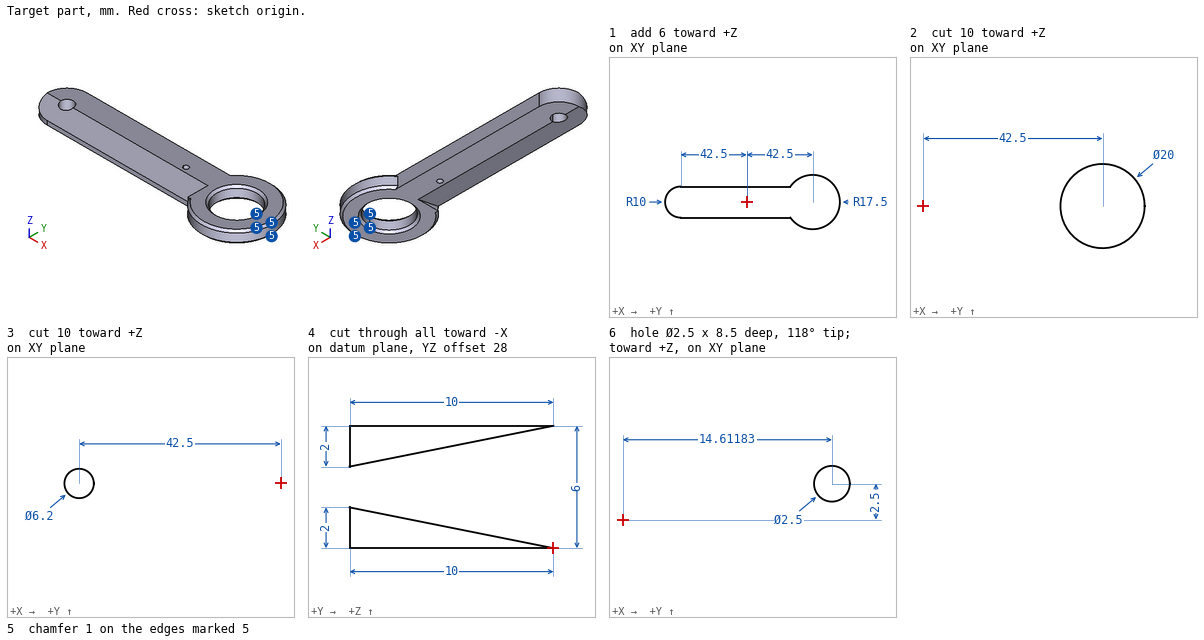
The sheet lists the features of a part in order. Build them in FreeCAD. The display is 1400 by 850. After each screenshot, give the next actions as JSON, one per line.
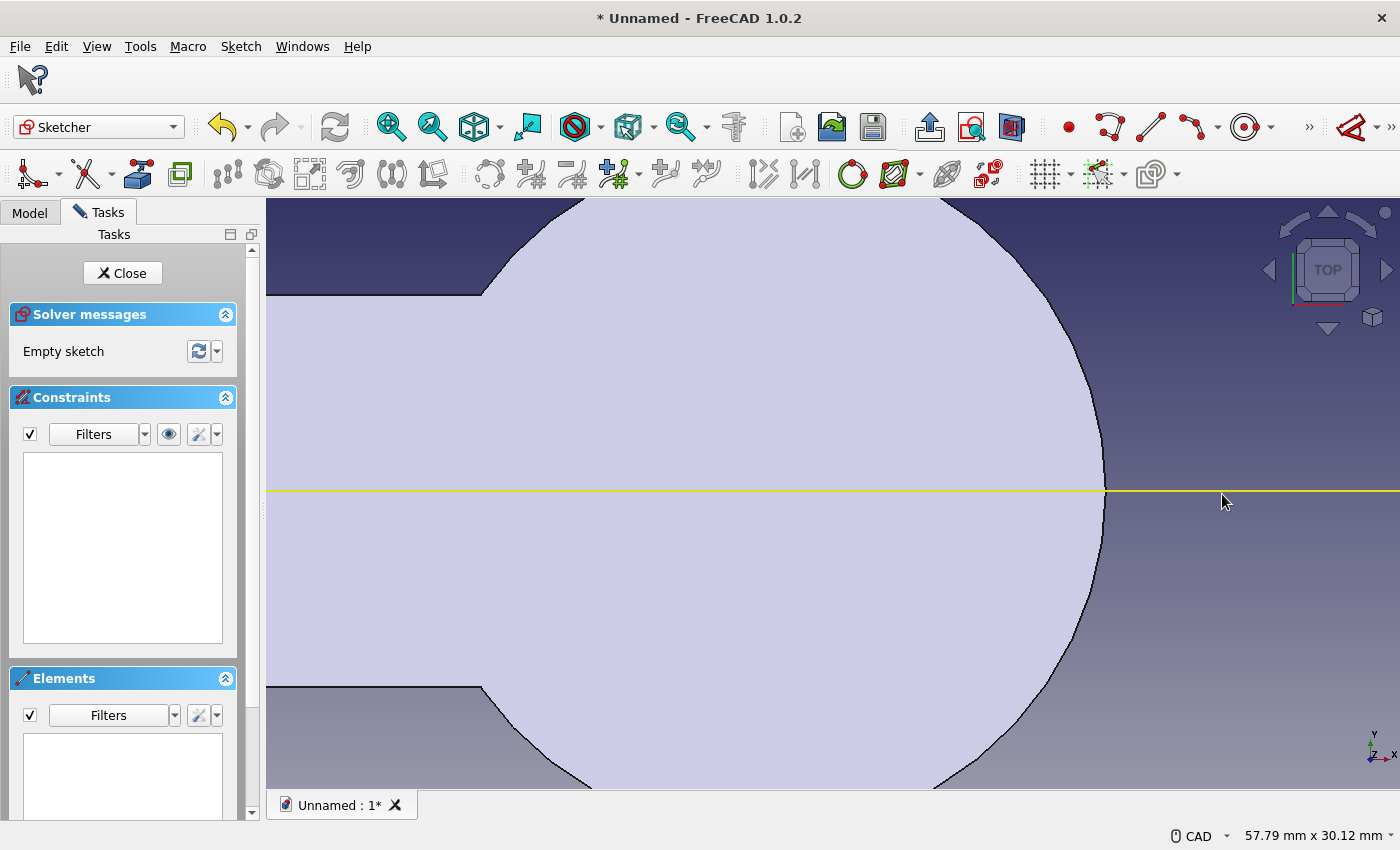
{"action": "key", "text": "g c"}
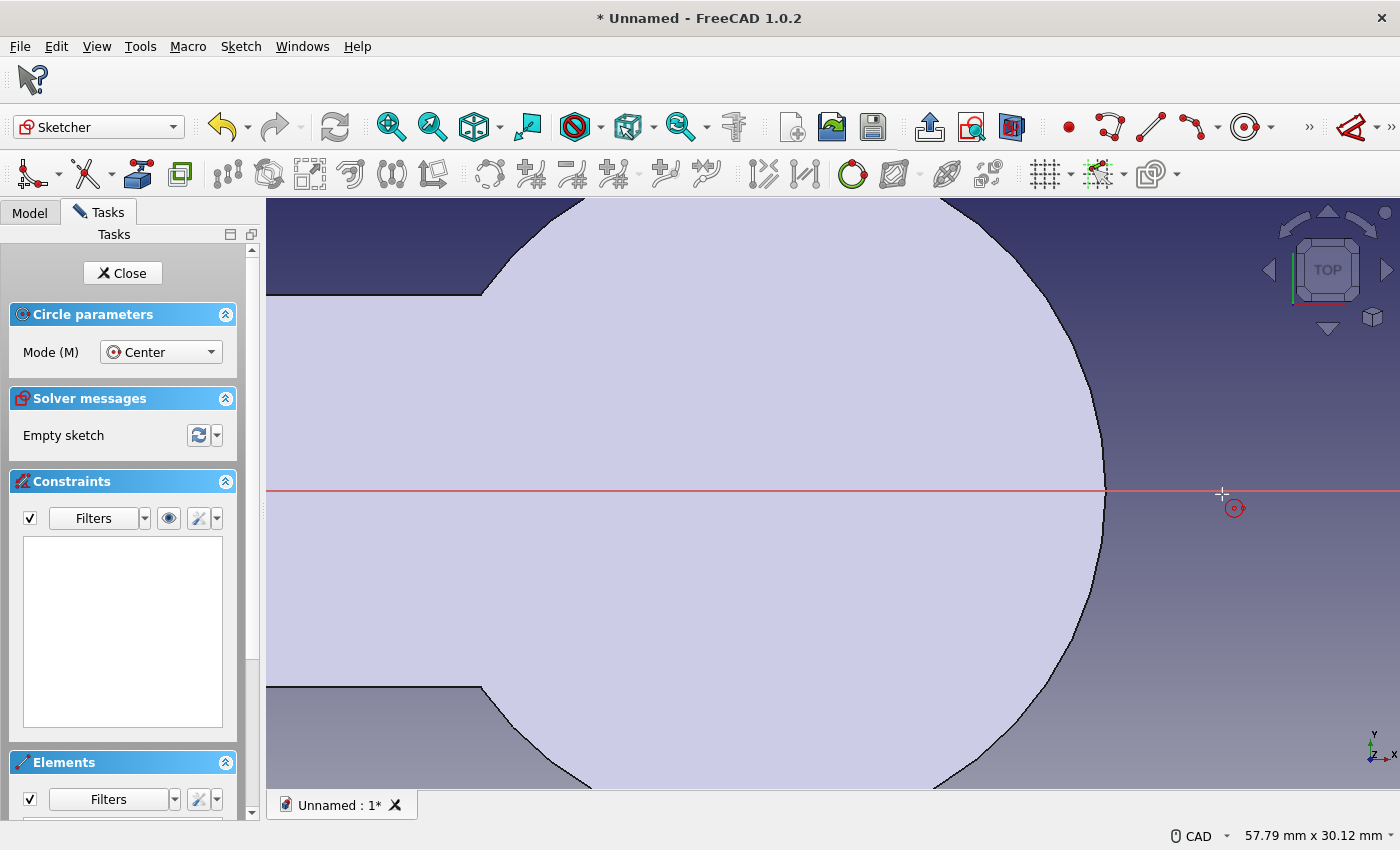
{"action": "left_click", "coordinate": [762, 491]}
{"action": "left_click", "coordinate": [901, 352]}
{"action": "key", "text": "Escape"}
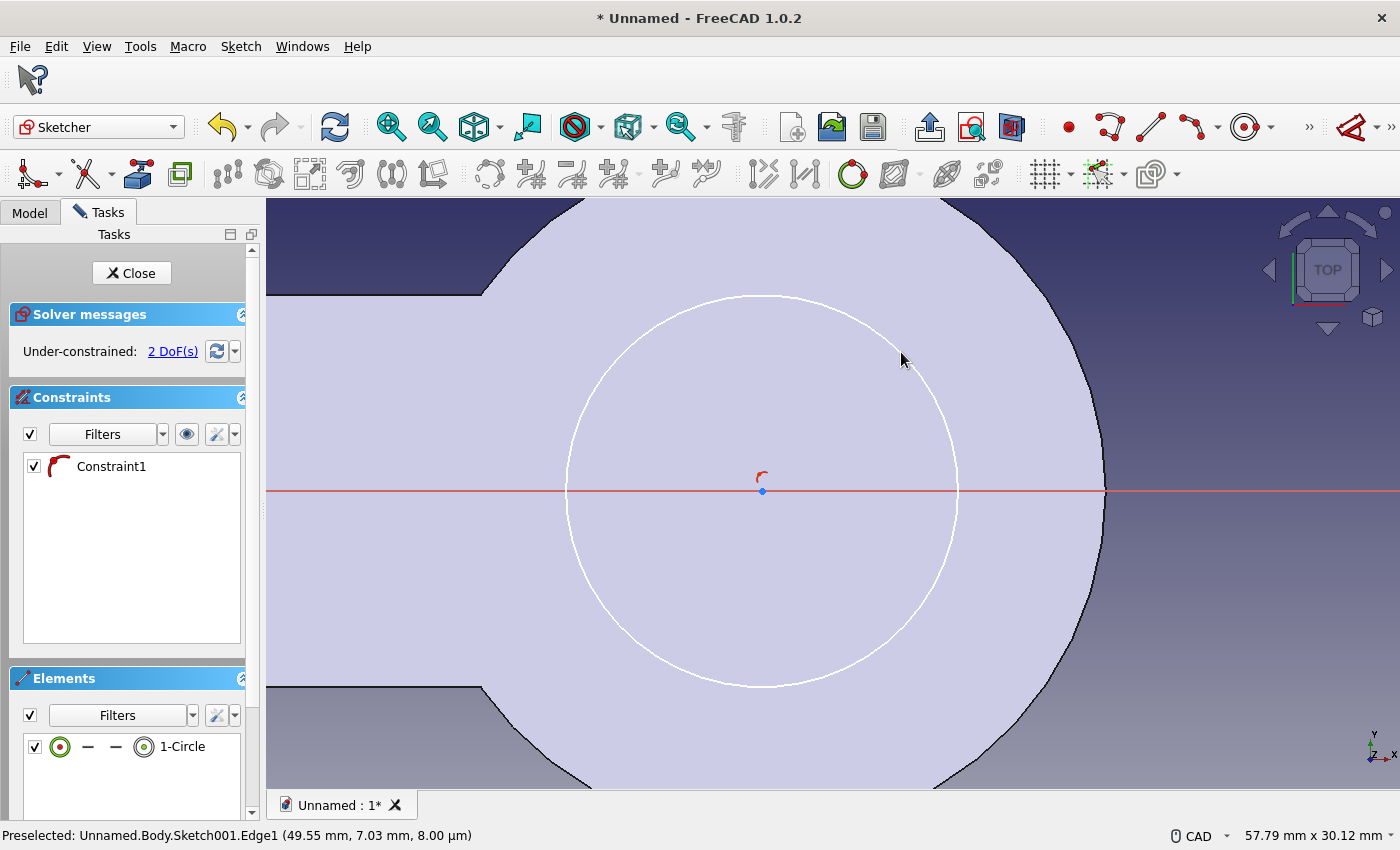
{"action": "left_click", "coordinate": [1350, 128]}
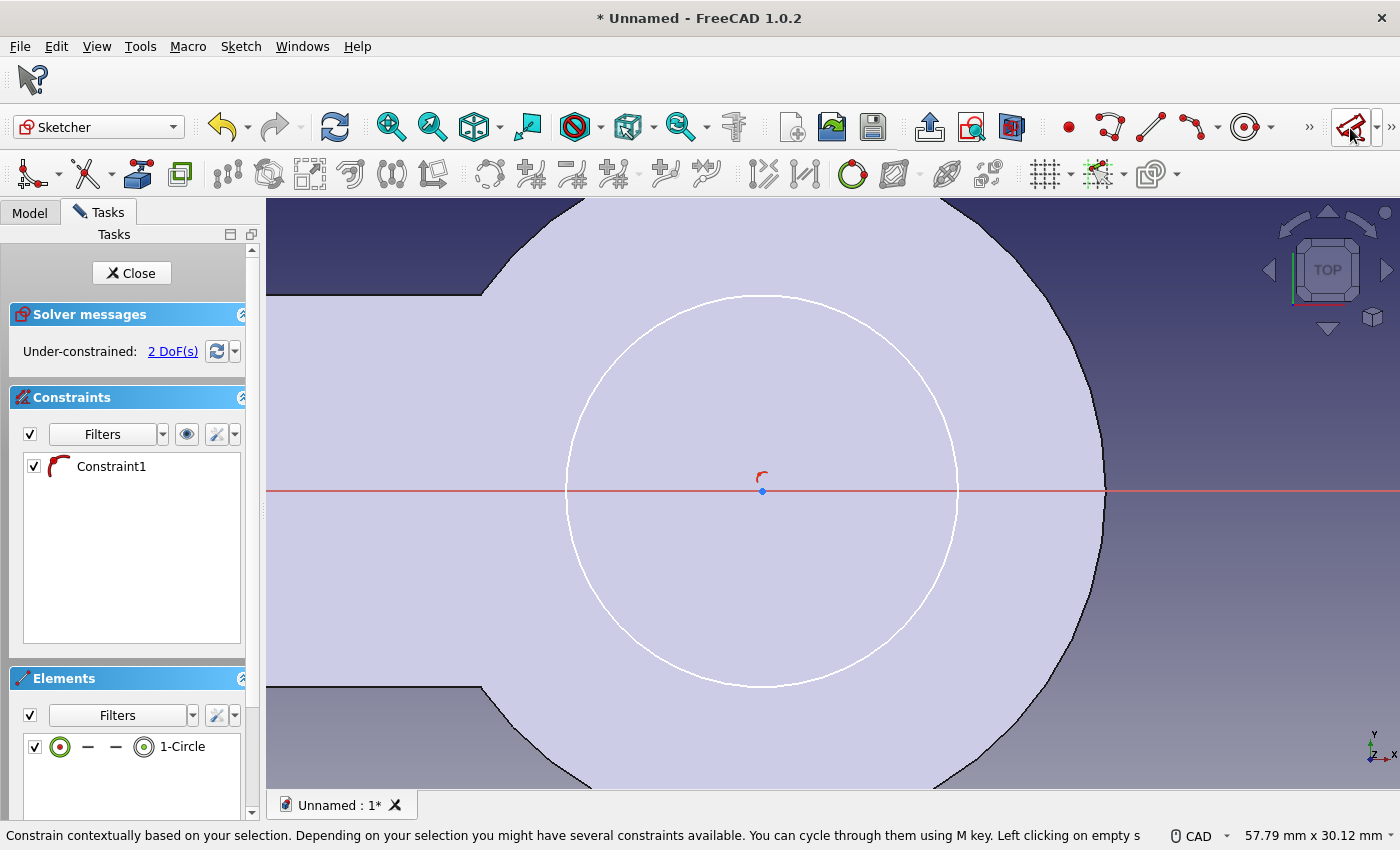
{"action": "left_click", "coordinate": [900, 352]}
{"action": "left_click", "coordinate": [923, 329]}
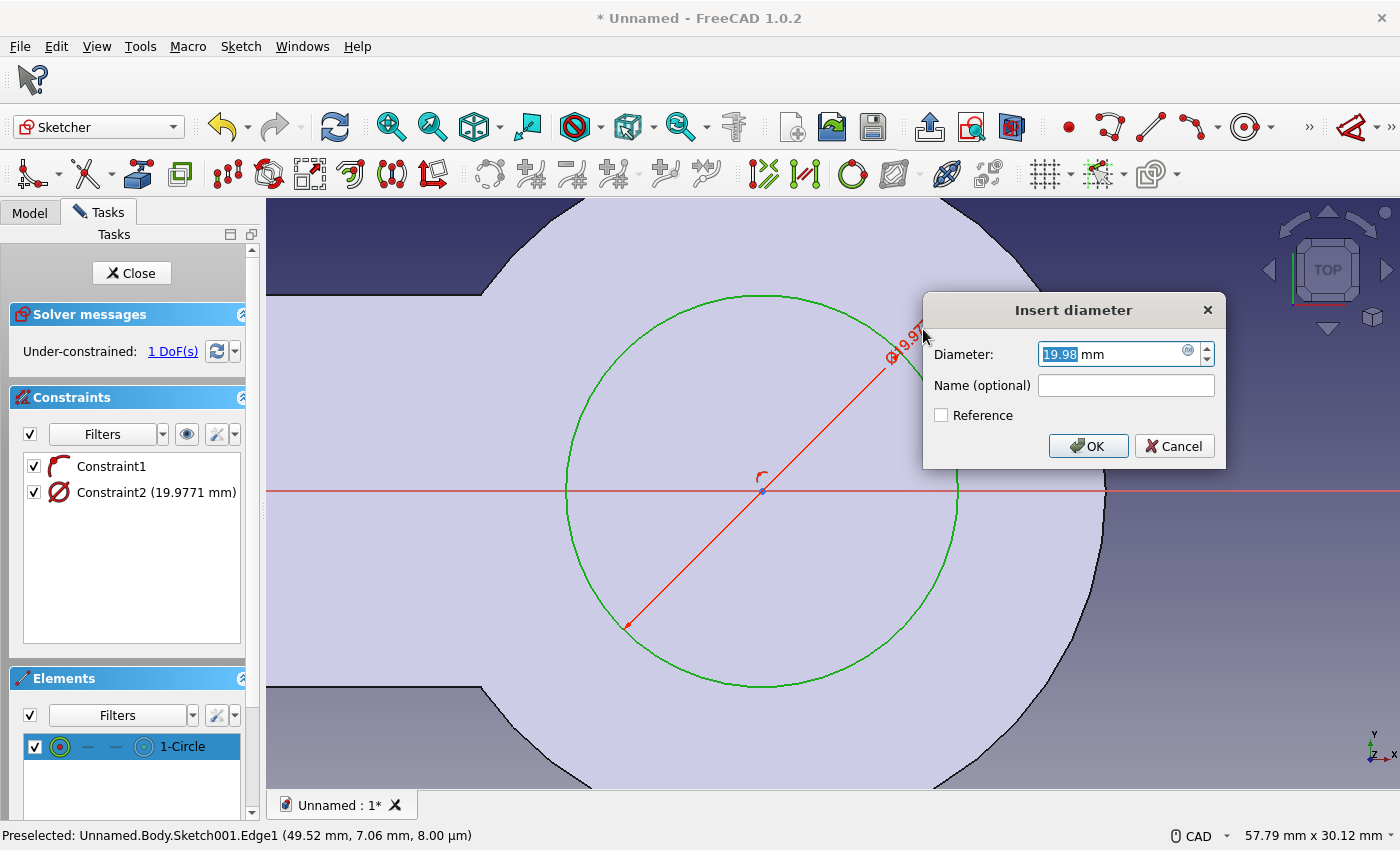
{"action": "type", "text": "20"}
{"action": "key", "text": "Return"}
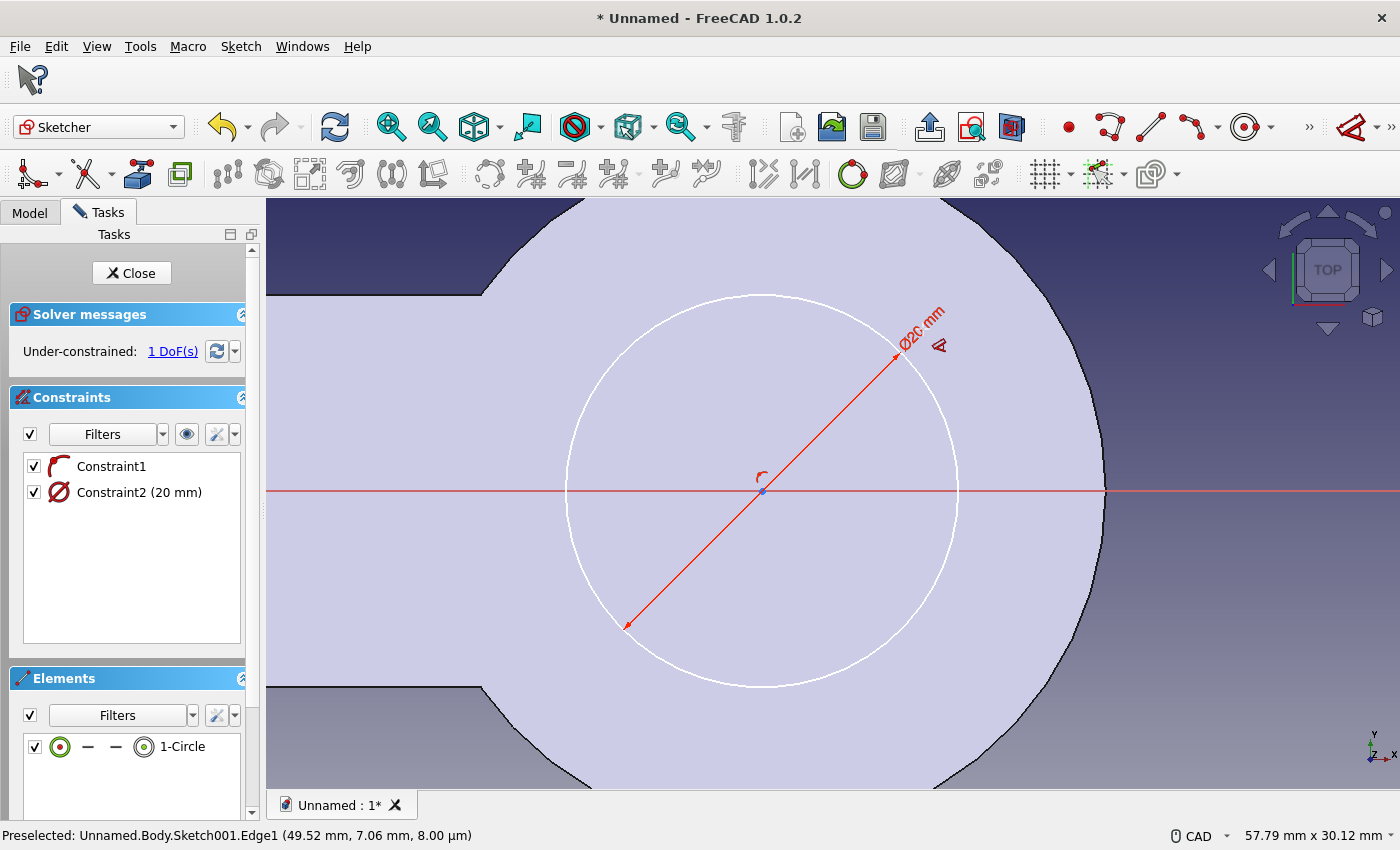
{"action": "left_click", "coordinate": [762, 491]}
{"action": "left_click", "coordinate": [528, 525]}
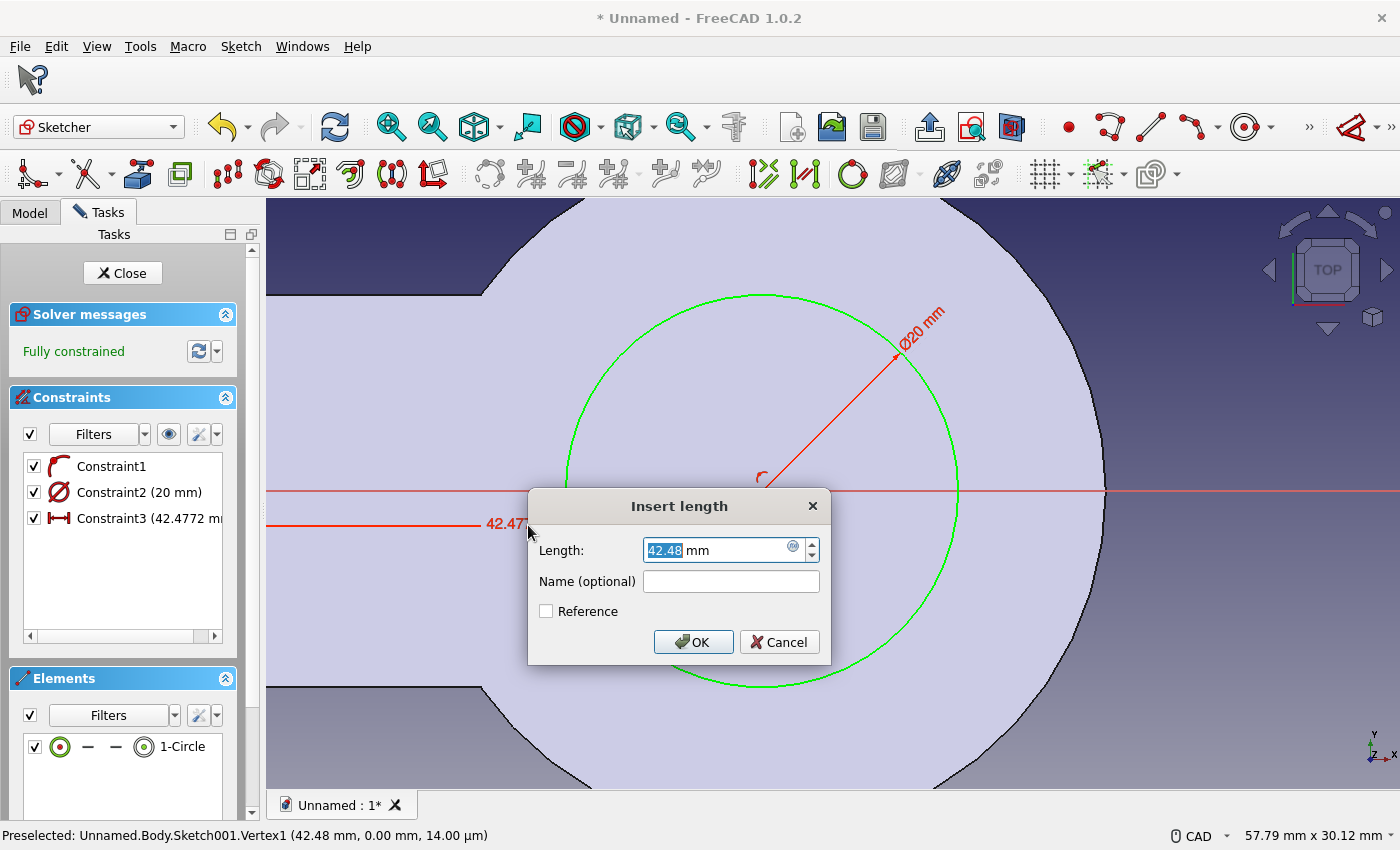
{"action": "type", "text": "42.5"}
{"action": "key", "text": "Return"}
{"action": "key", "text": "Escape"}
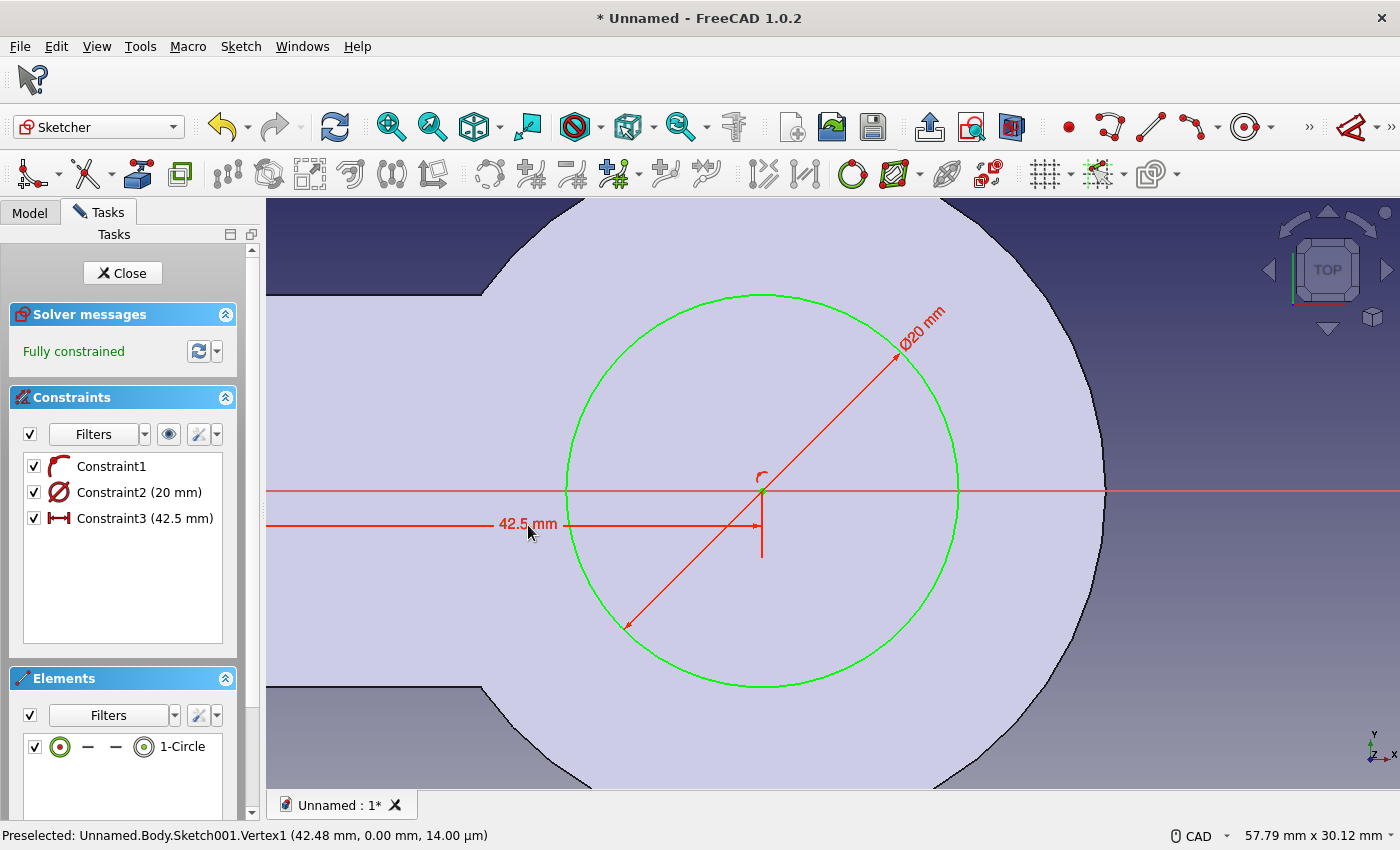
{"action": "left_click", "coordinate": [123, 273]}